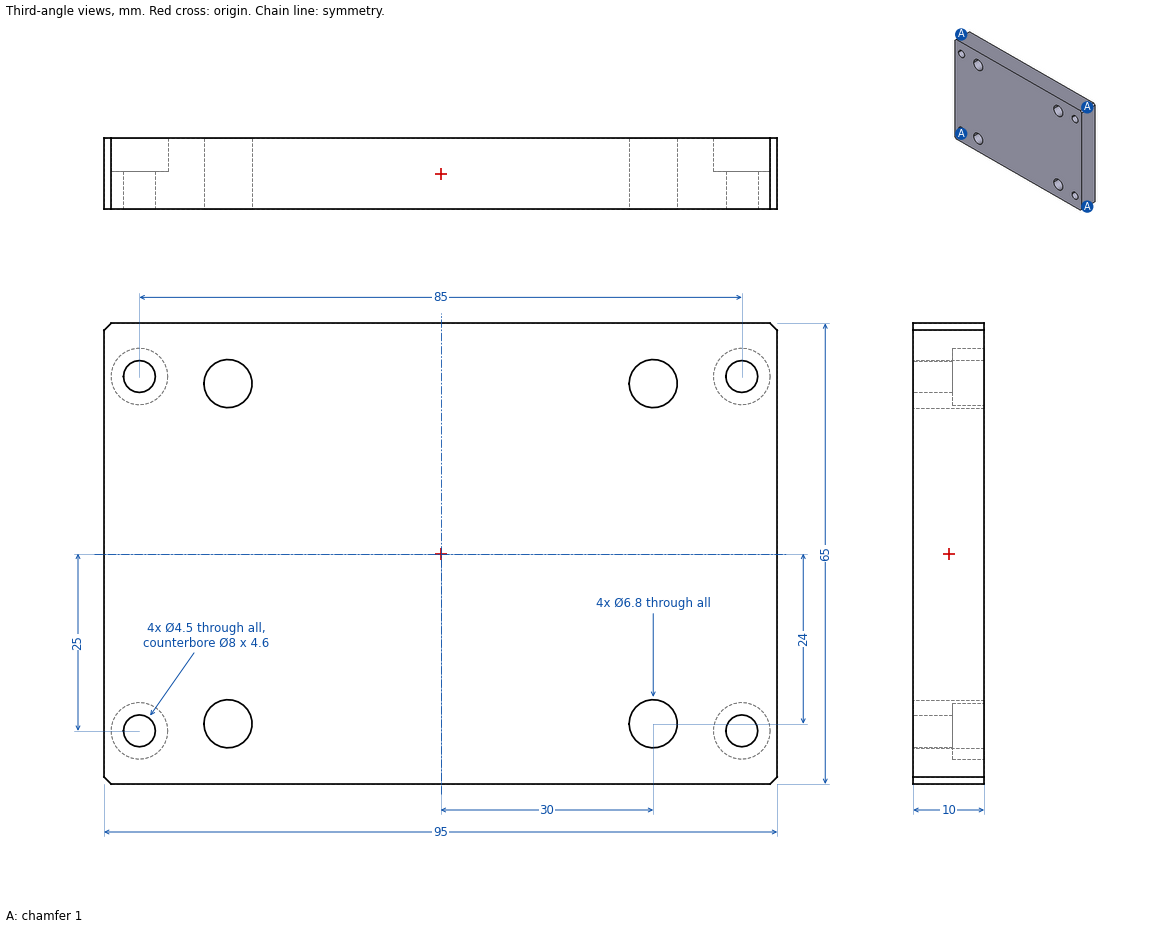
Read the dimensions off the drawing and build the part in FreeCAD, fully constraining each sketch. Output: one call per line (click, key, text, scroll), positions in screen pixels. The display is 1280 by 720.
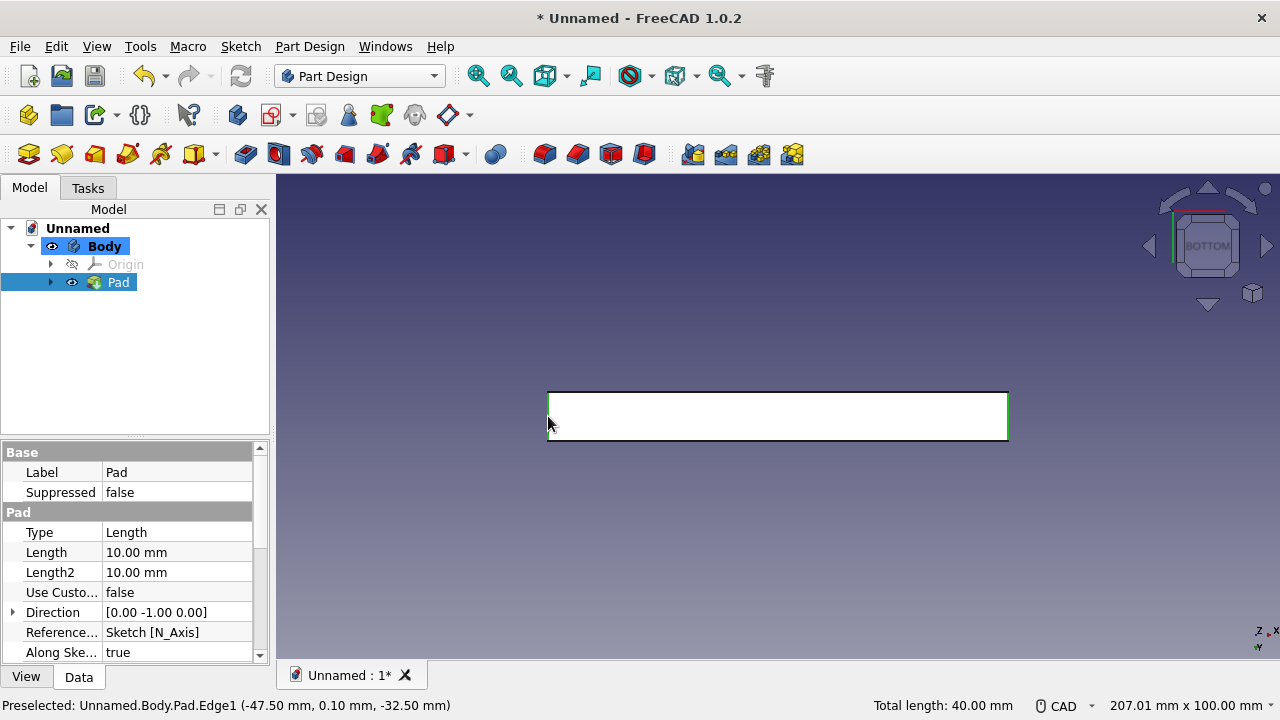
click(578, 154)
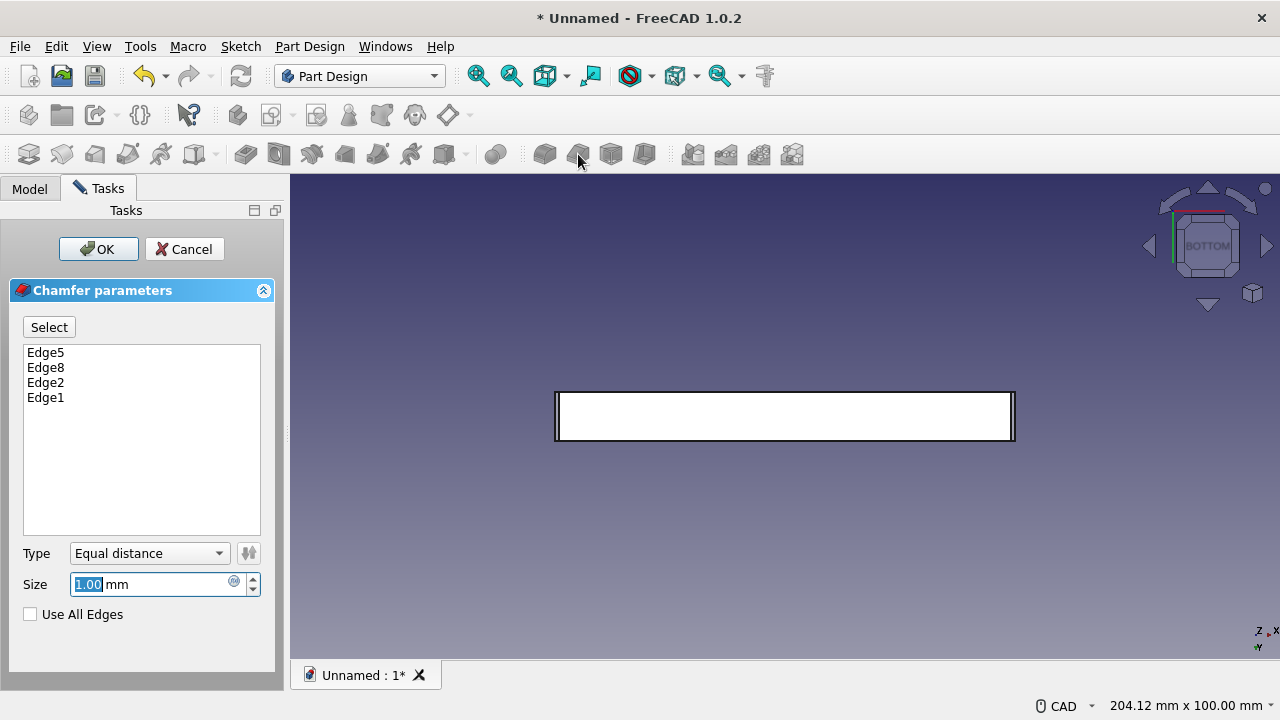
text(1)
key(Tab)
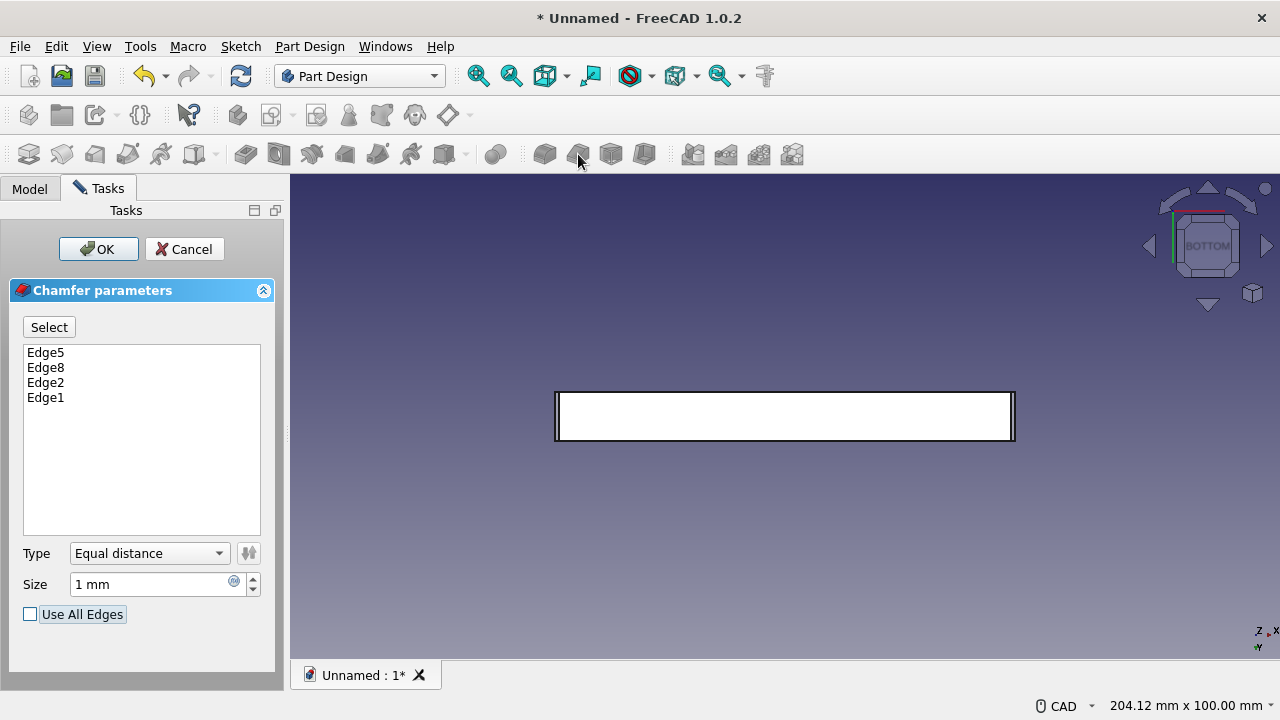
click(99, 249)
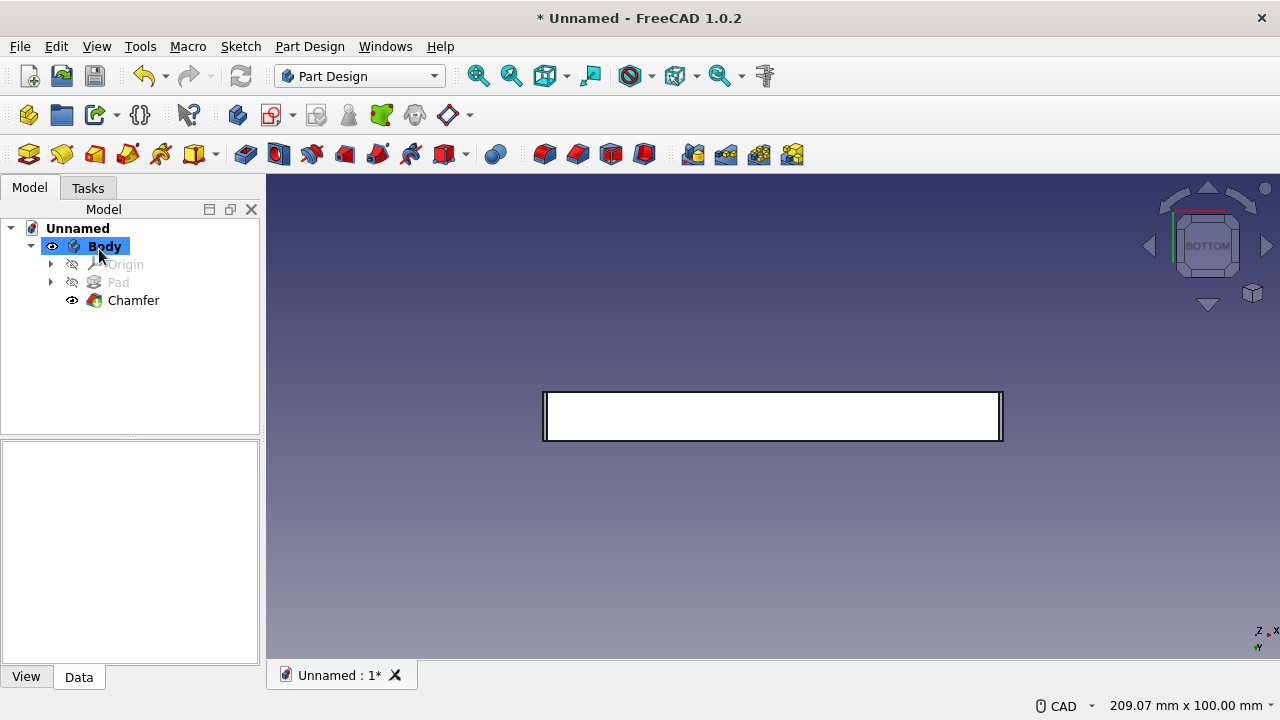
key(4)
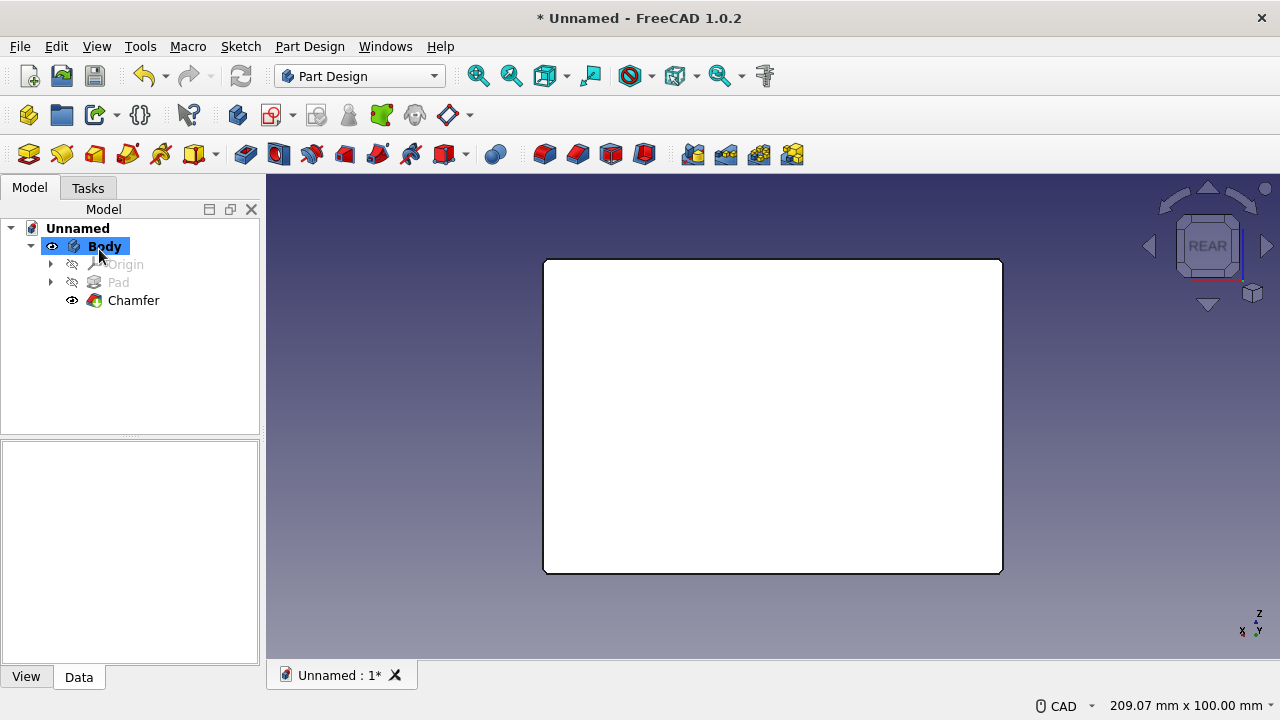
click(707, 415)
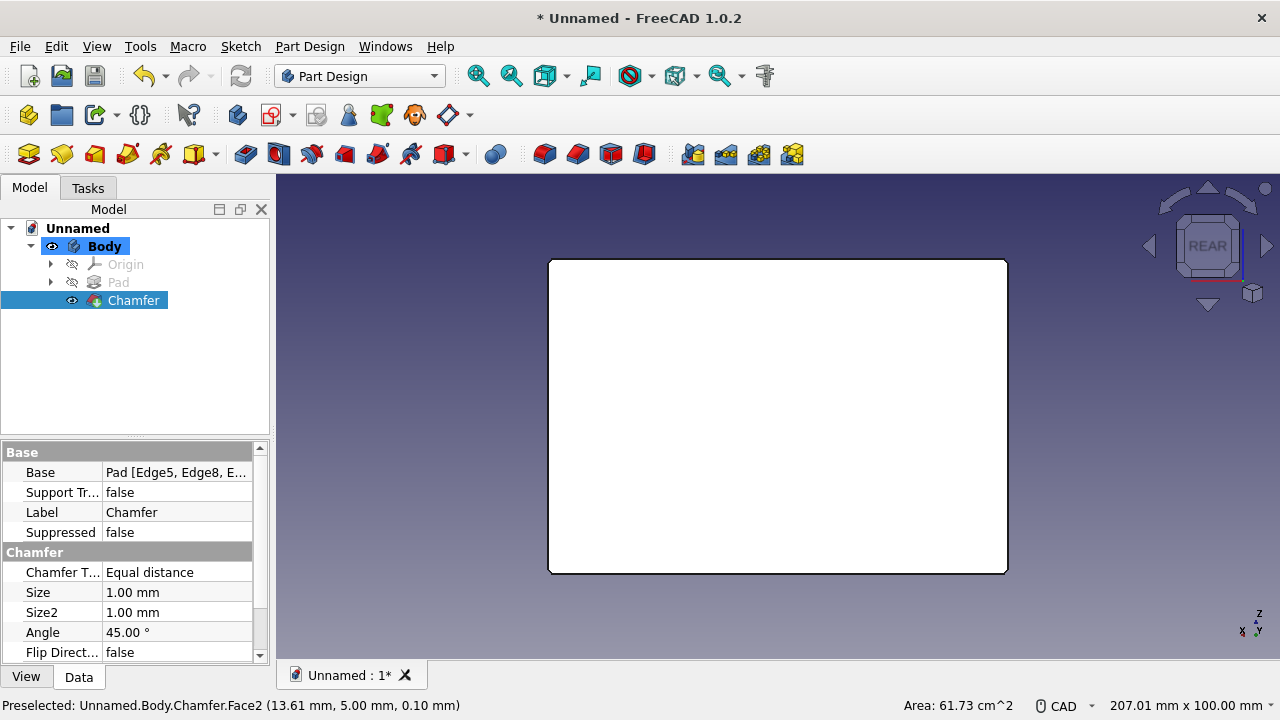
click(270, 116)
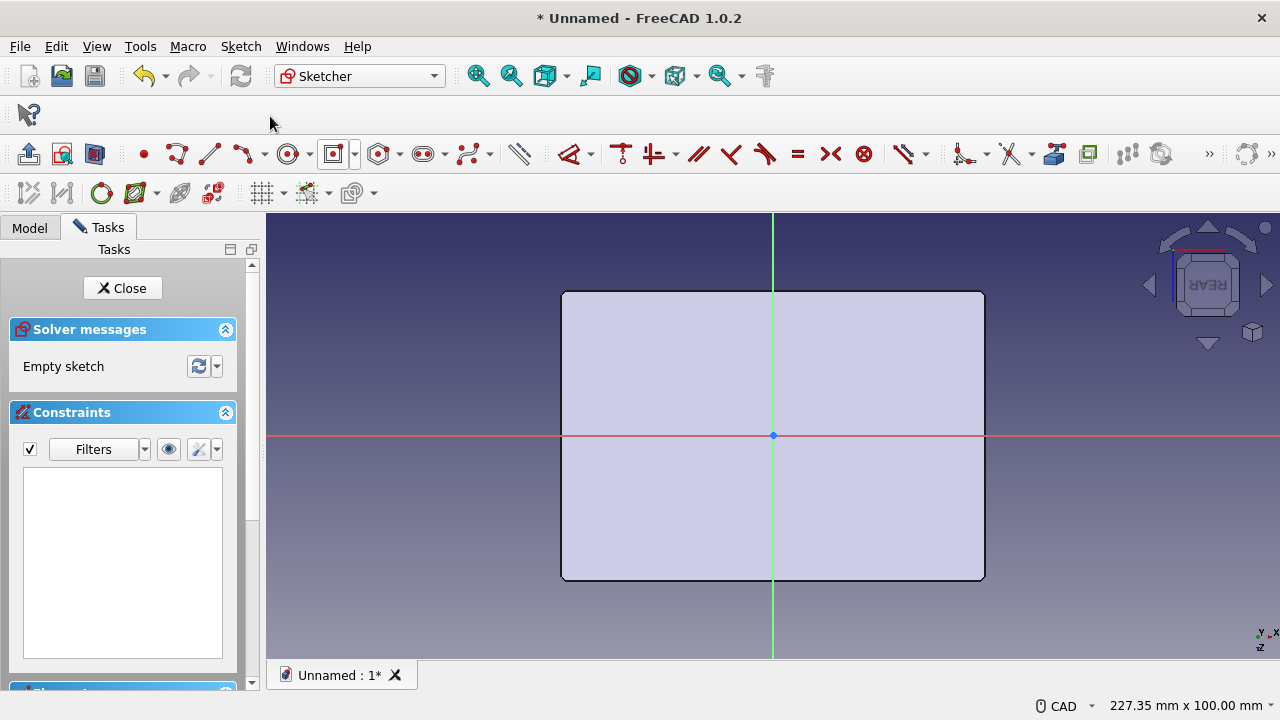
click(288, 154)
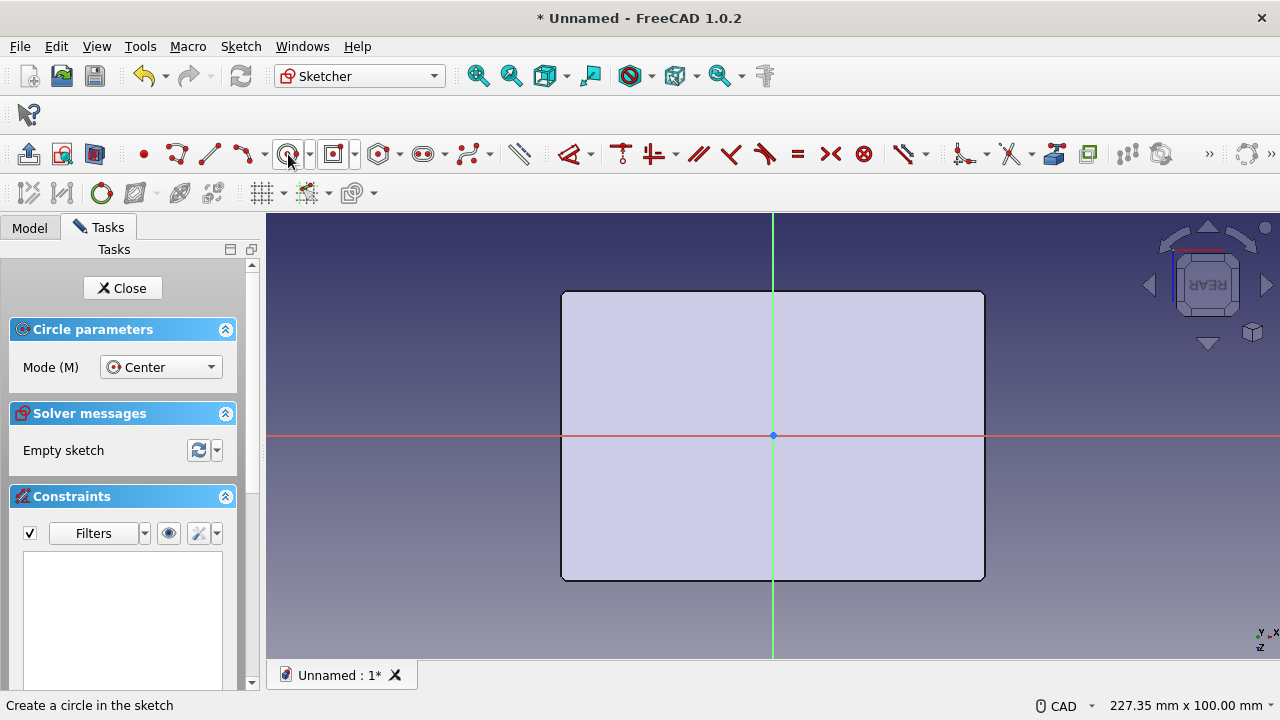
scroll(583, 325, up, 5)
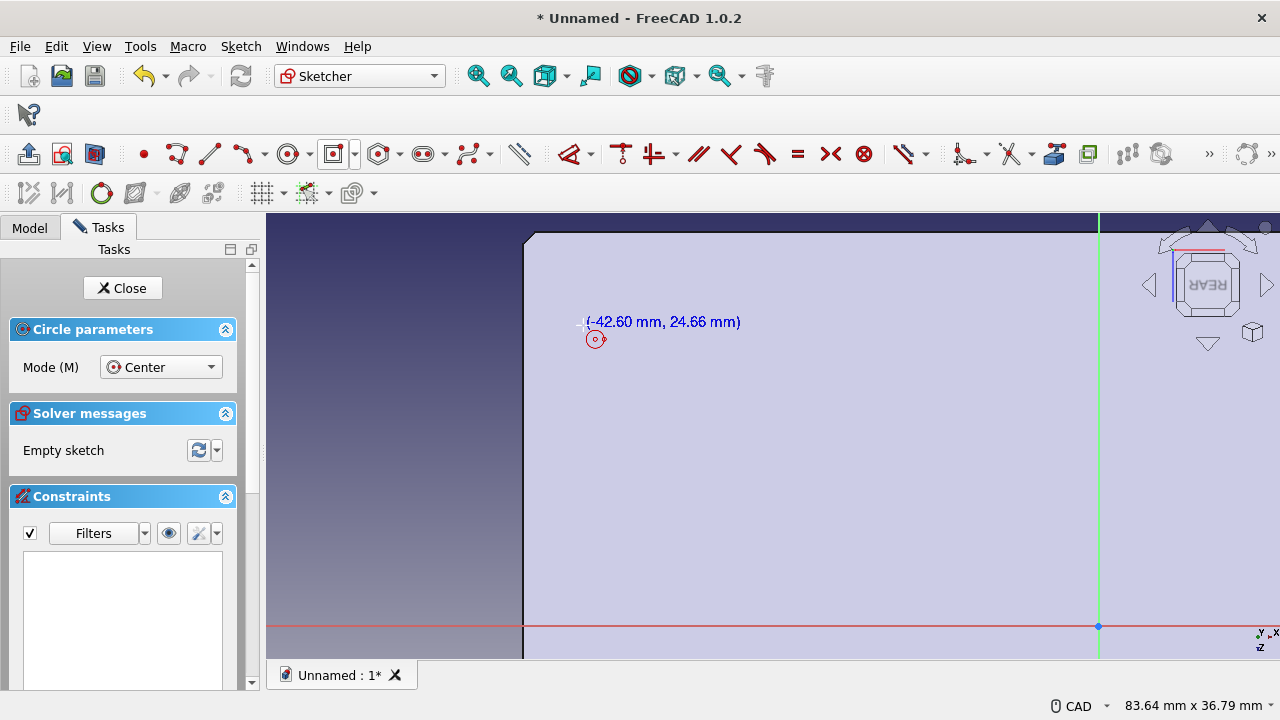
click(584, 323)
move(603, 304)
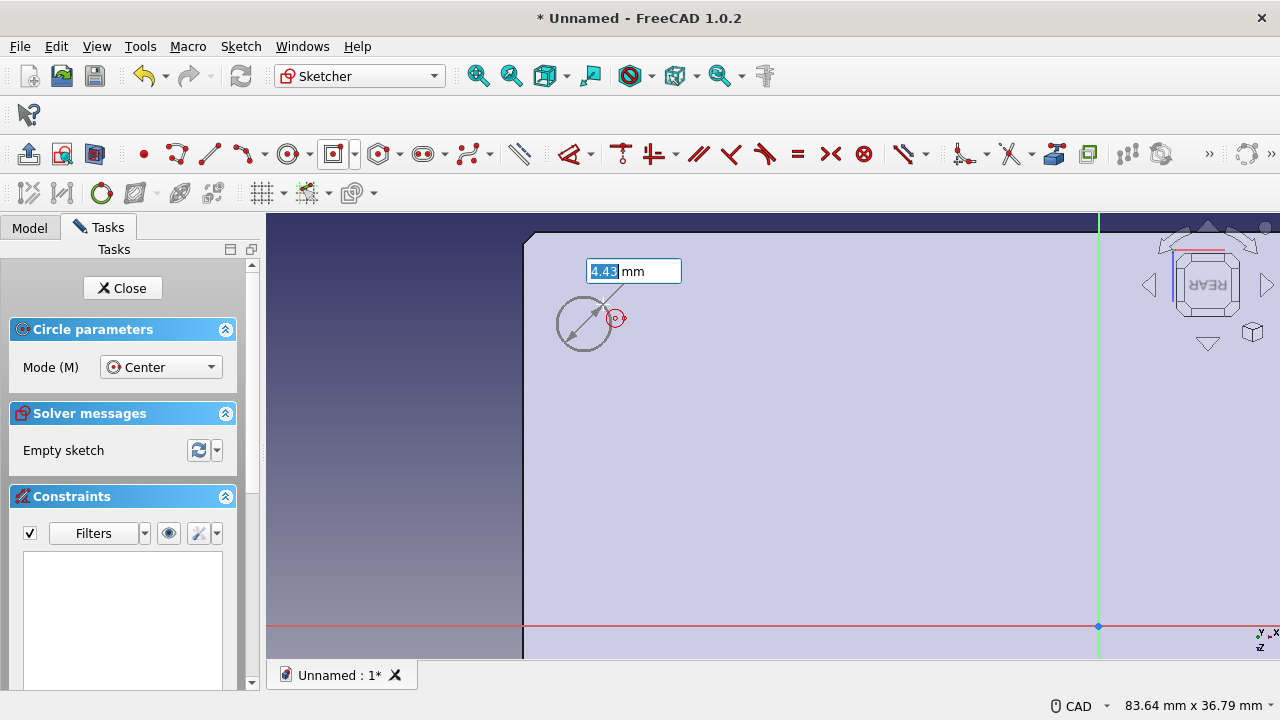
text(4.5)
key(Return)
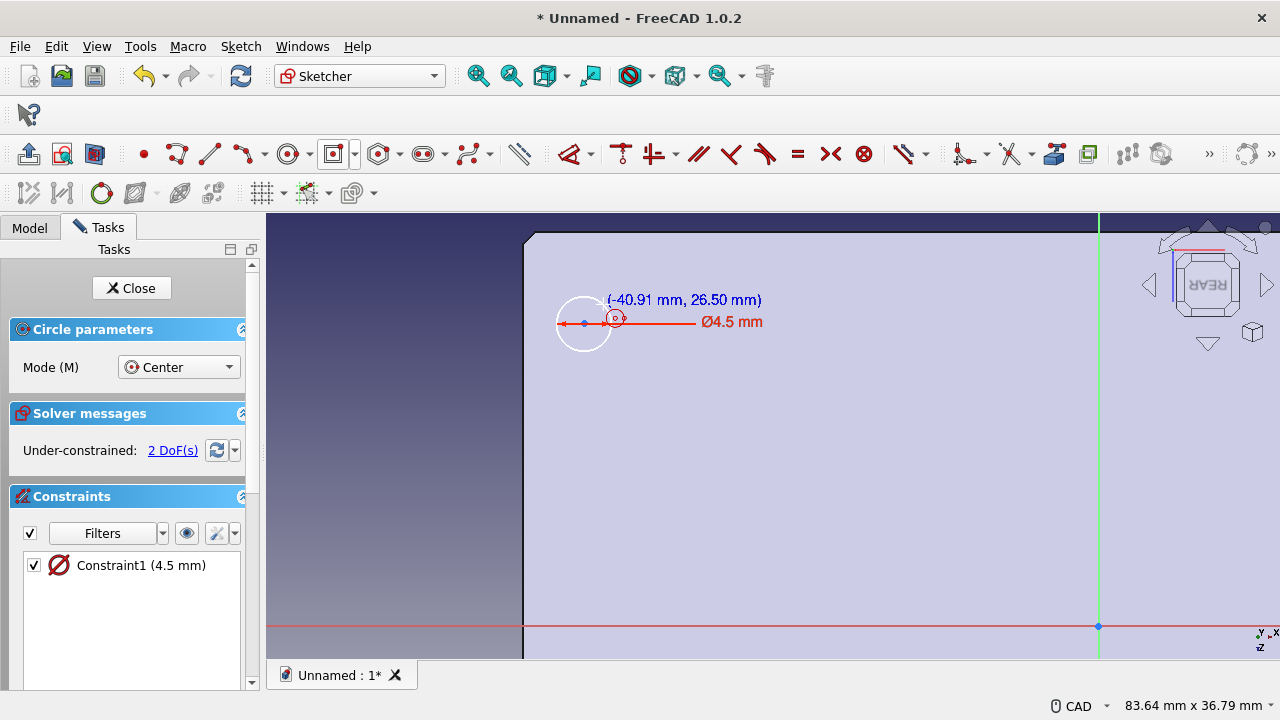
scroll(383, 281, down, 4)